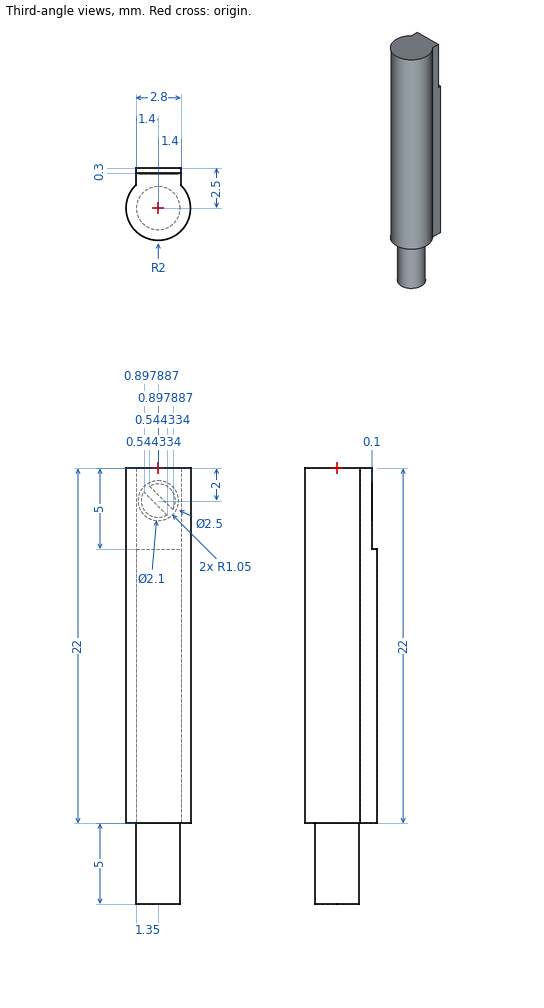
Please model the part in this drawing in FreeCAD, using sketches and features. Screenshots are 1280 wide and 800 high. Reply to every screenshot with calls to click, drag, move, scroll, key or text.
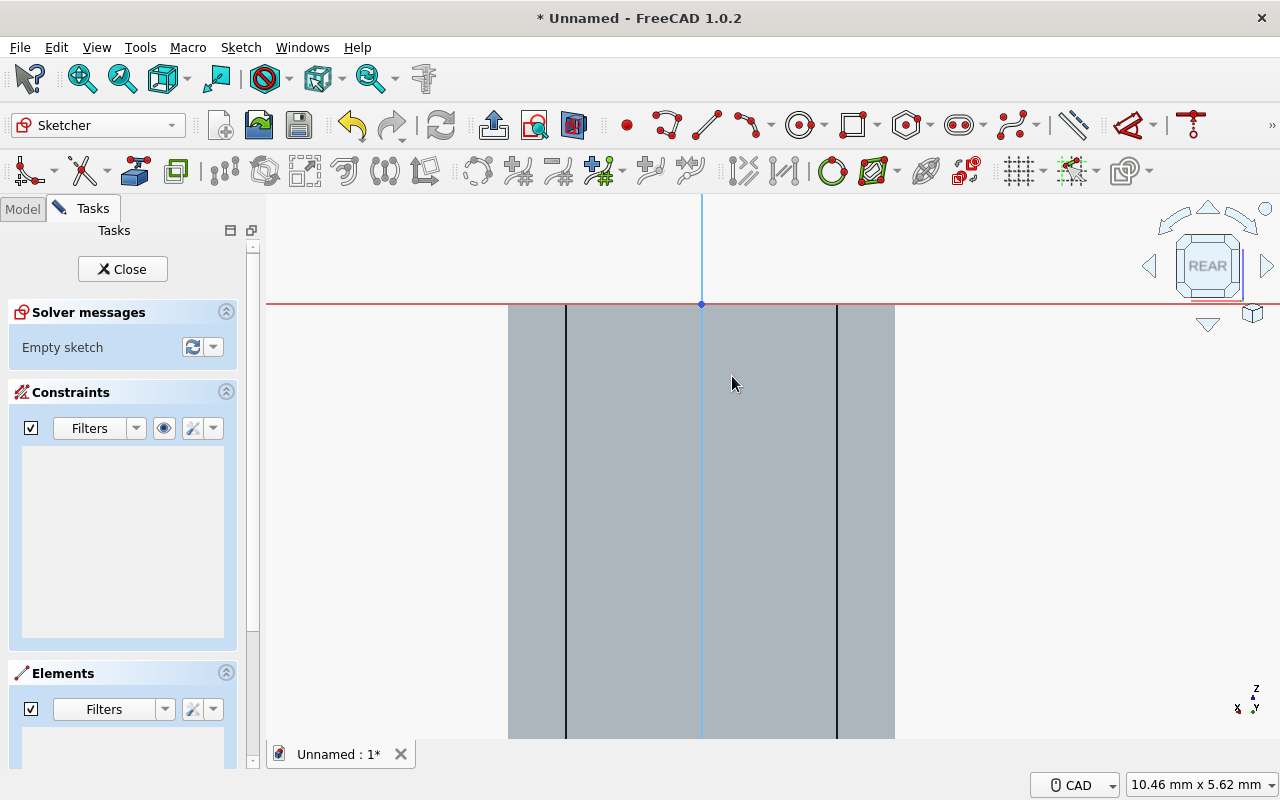
click(800, 126)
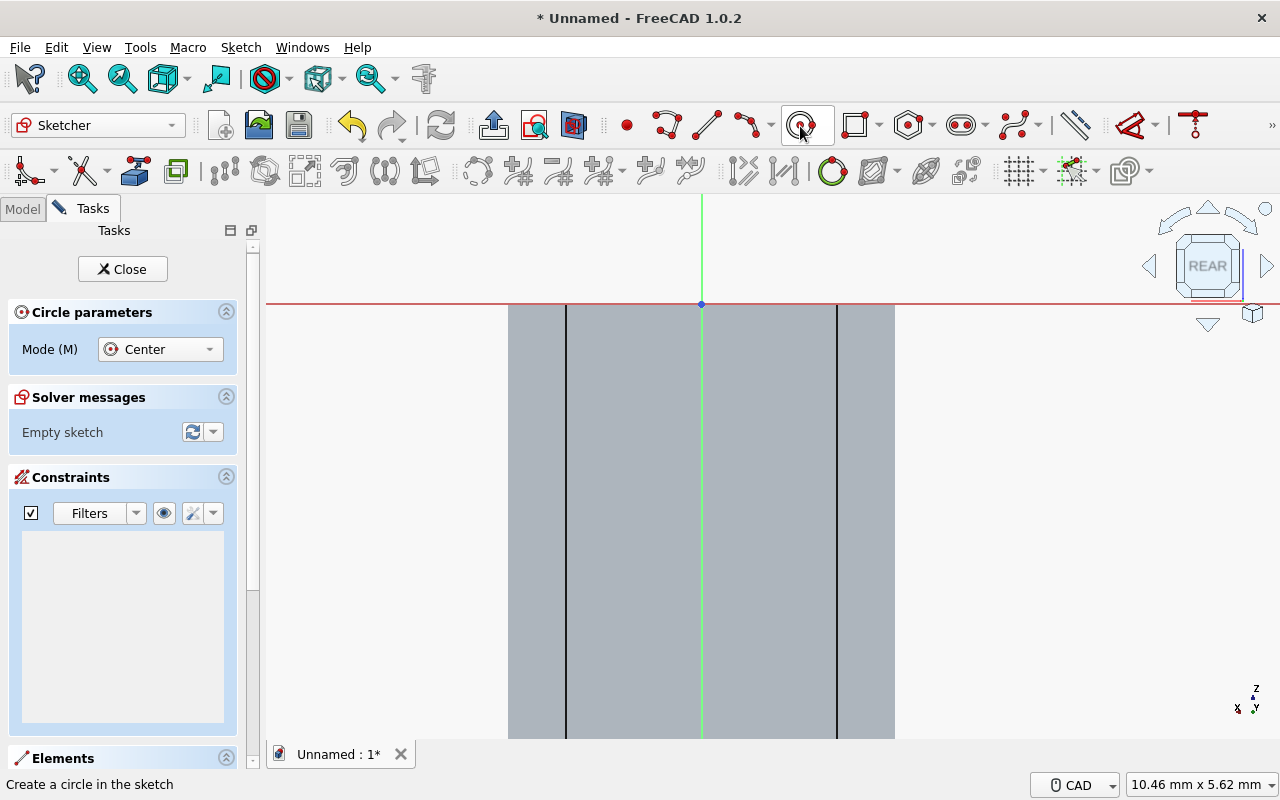
click(702, 498)
click(787, 413)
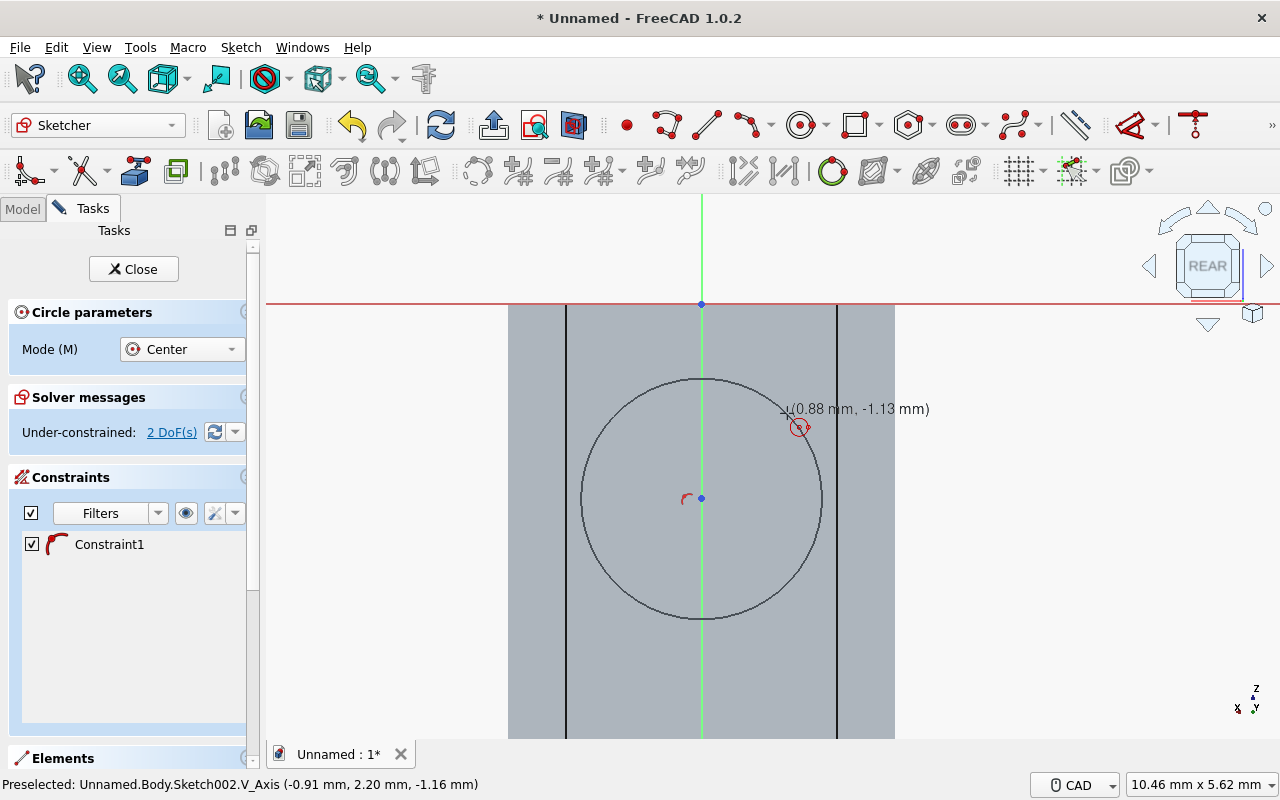
click(702, 499)
click(774, 426)
key(Escape)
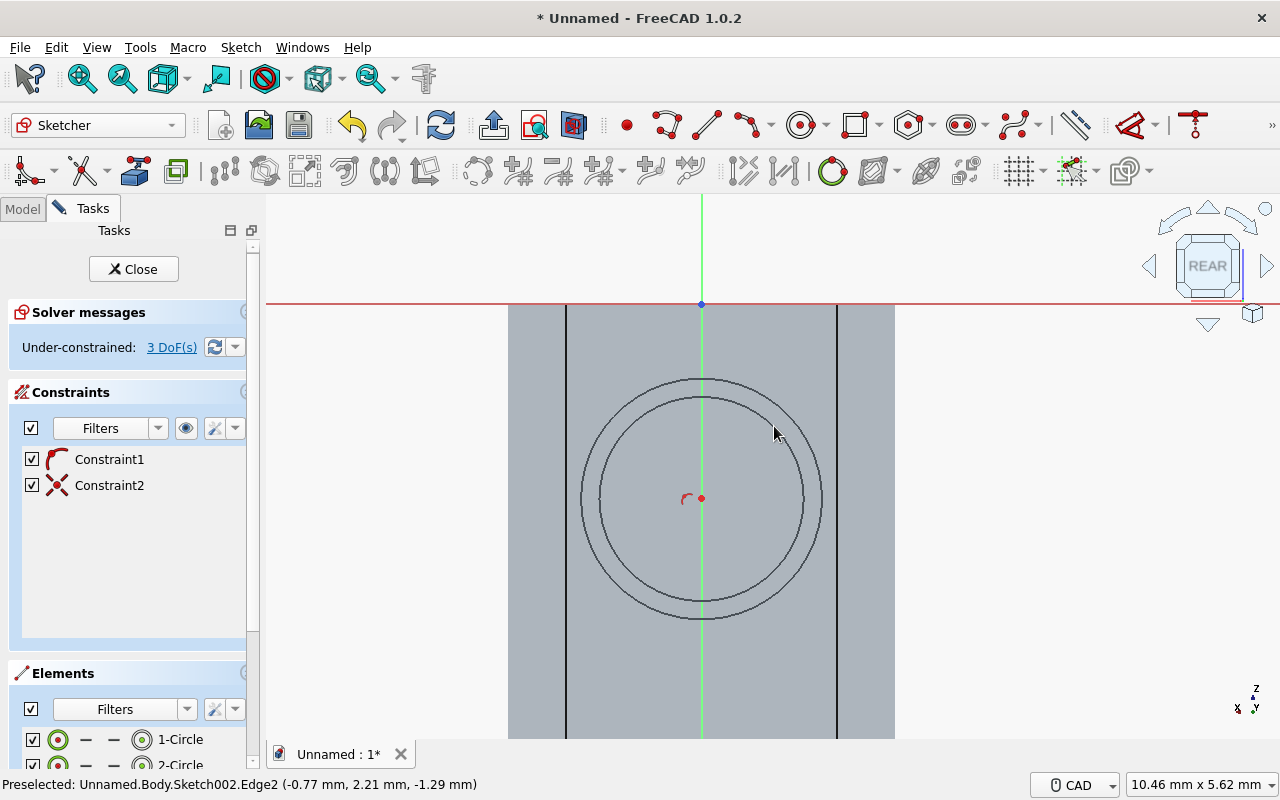
click(1130, 126)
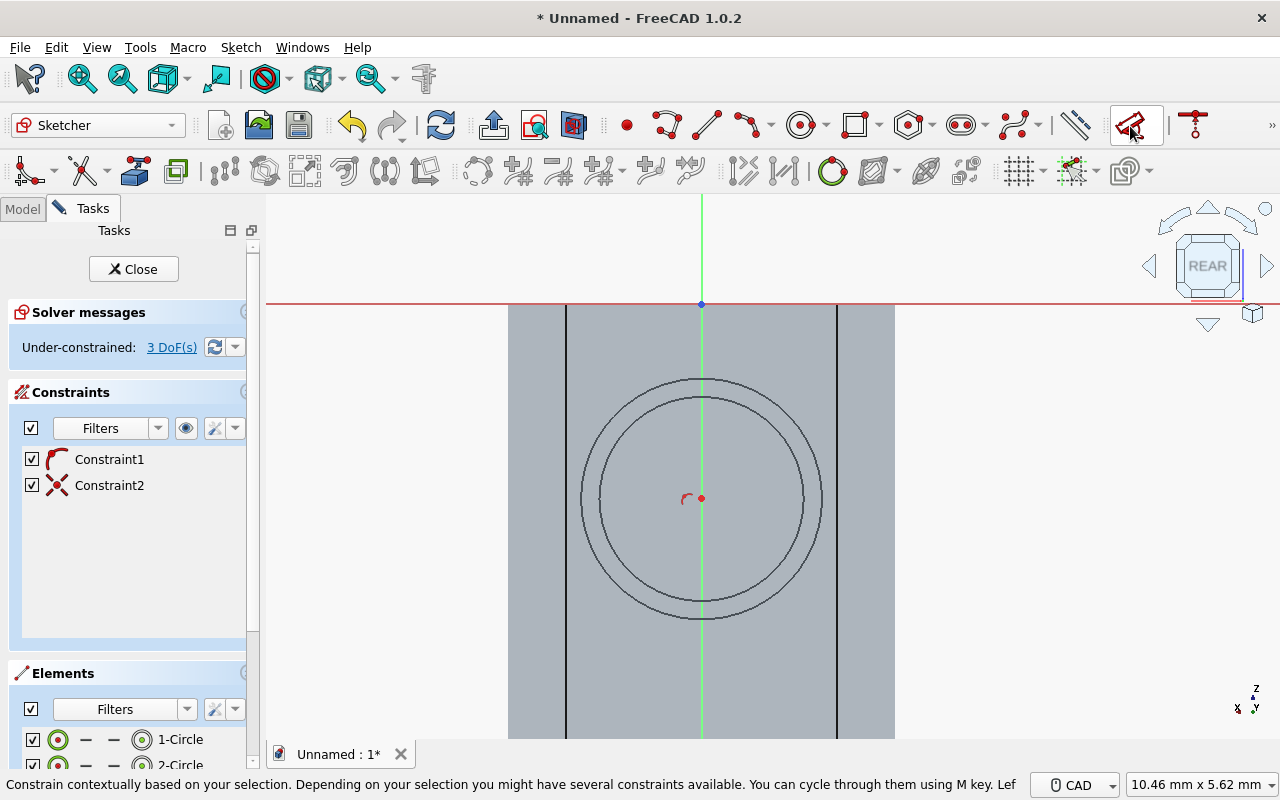
click(787, 414)
click(810, 391)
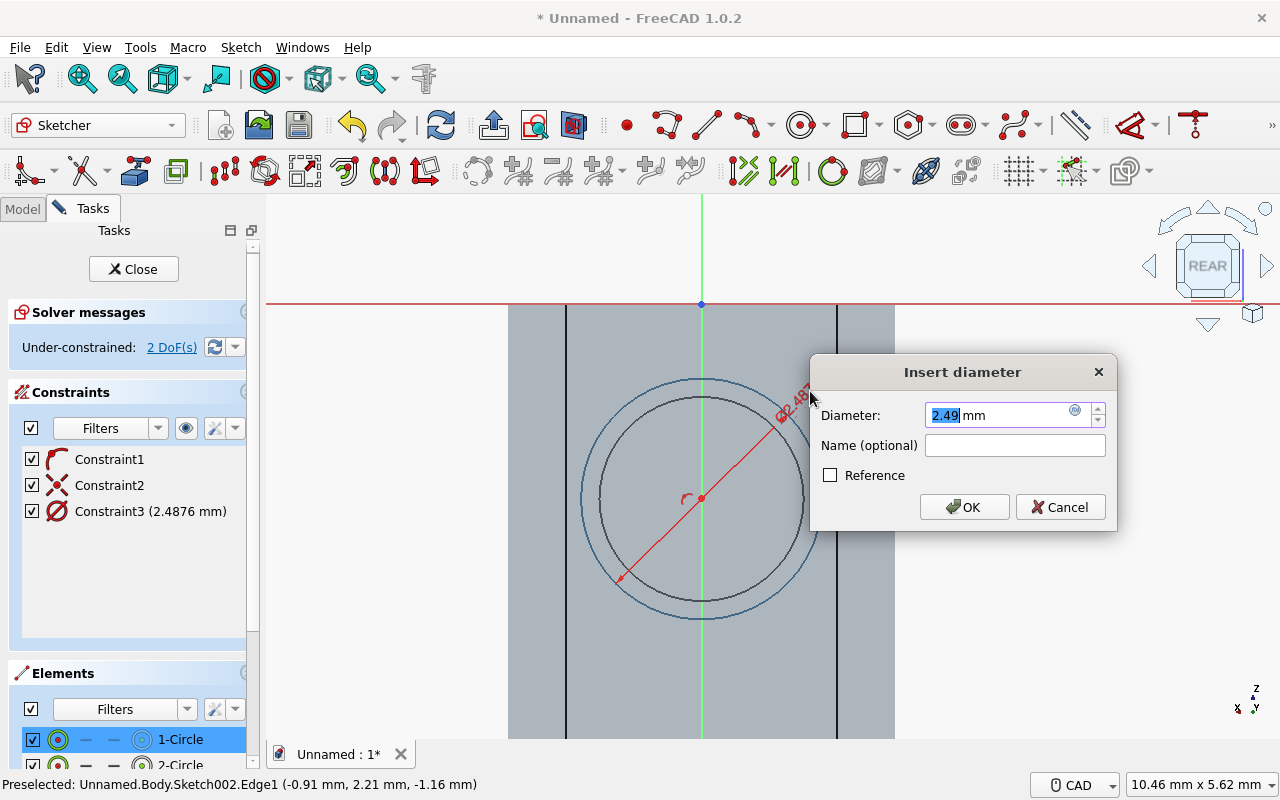
text(2.5)
key(Return)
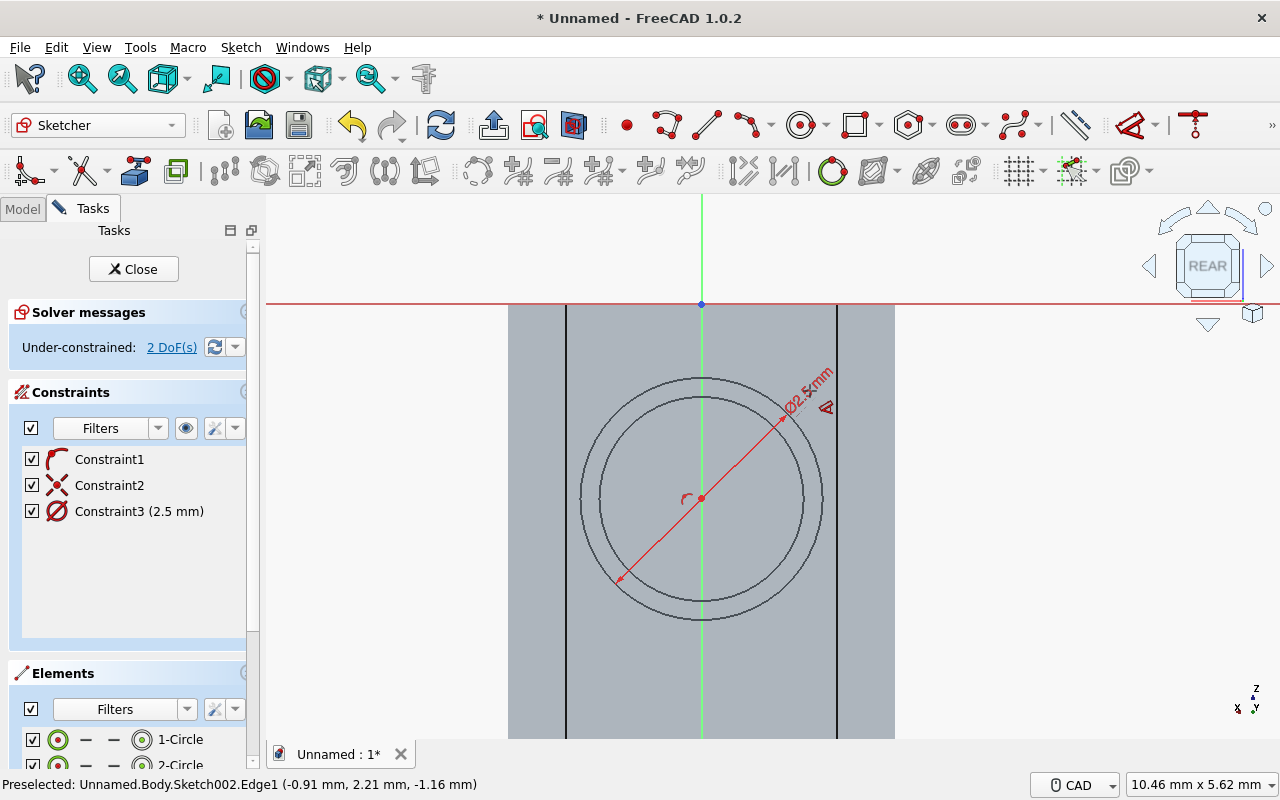
click(774, 427)
click(830, 462)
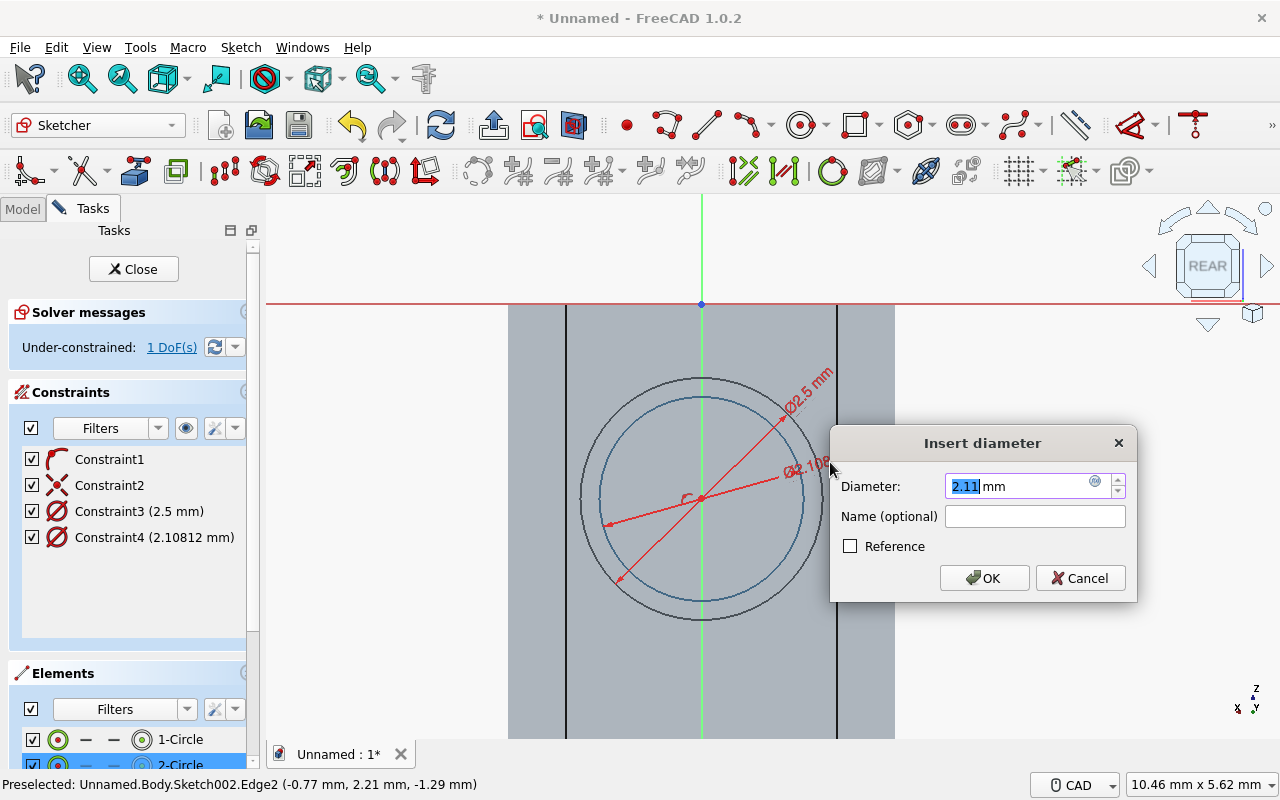
text(2.1)
key(Return)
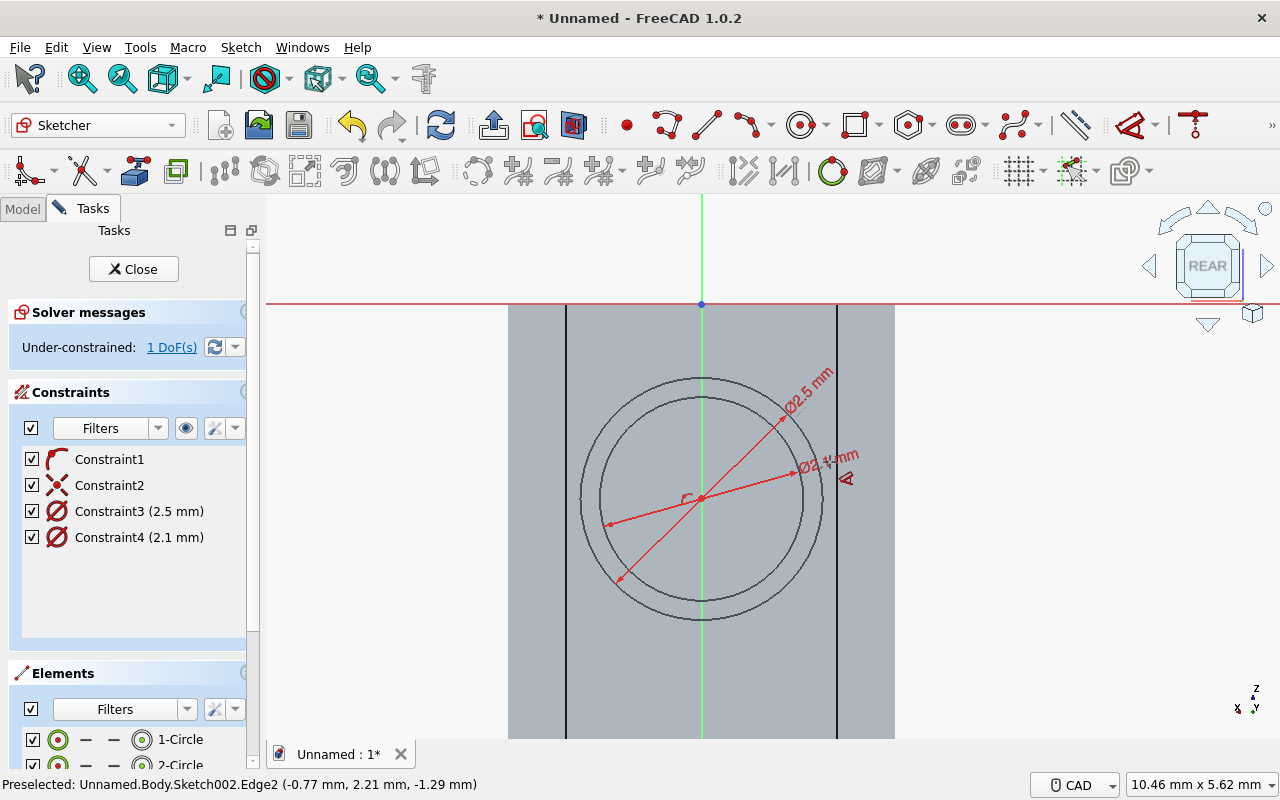
click(702, 499)
click(736, 357)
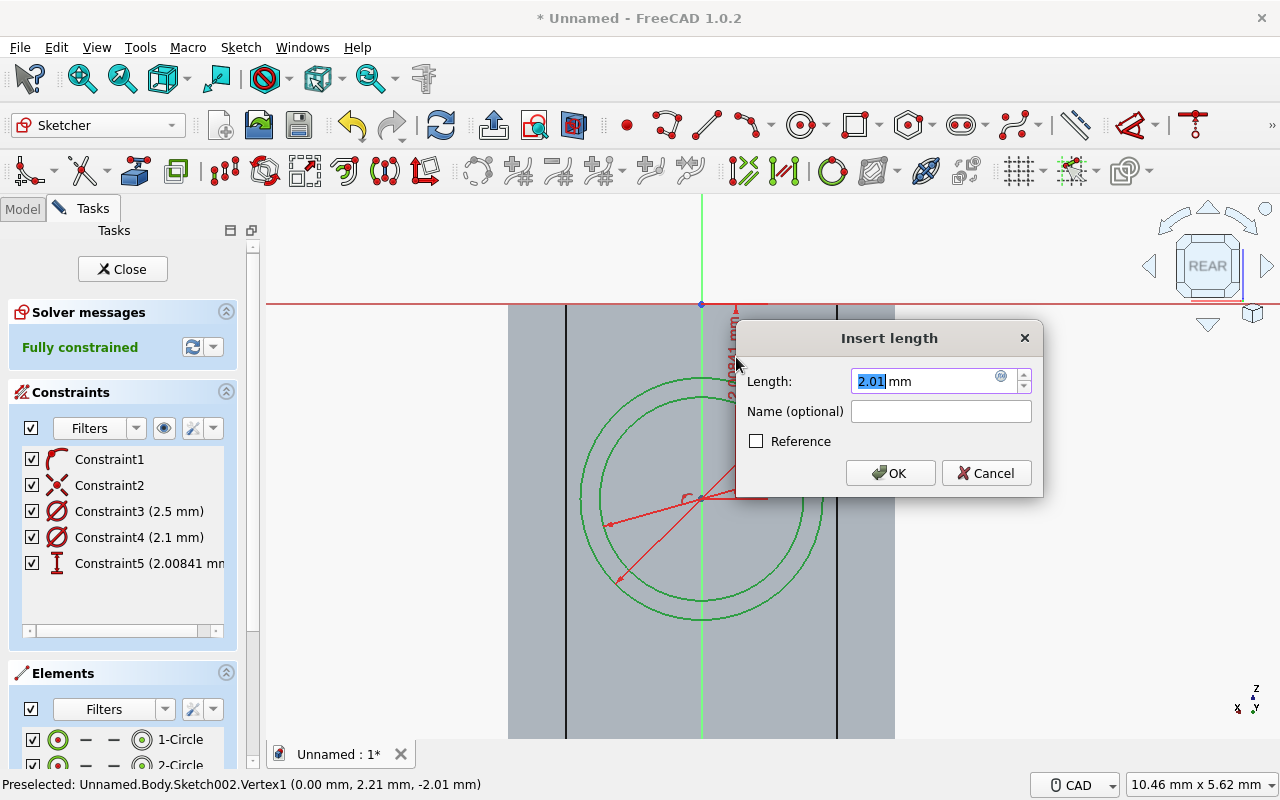
text(2)
key(Return)
key(Escape)